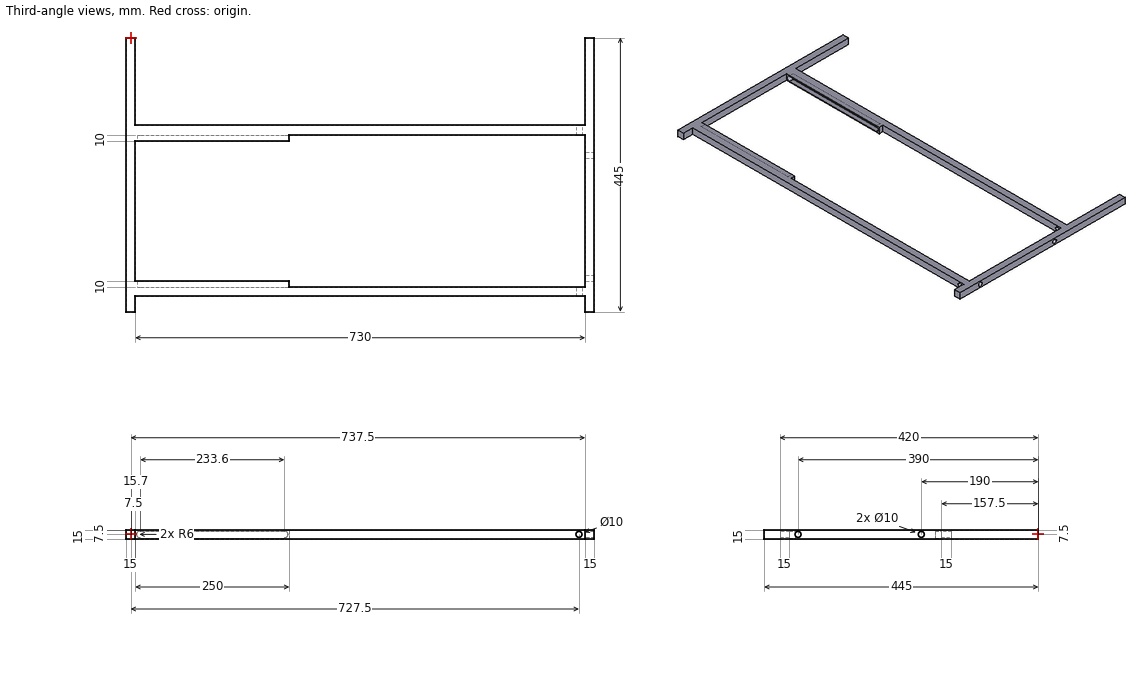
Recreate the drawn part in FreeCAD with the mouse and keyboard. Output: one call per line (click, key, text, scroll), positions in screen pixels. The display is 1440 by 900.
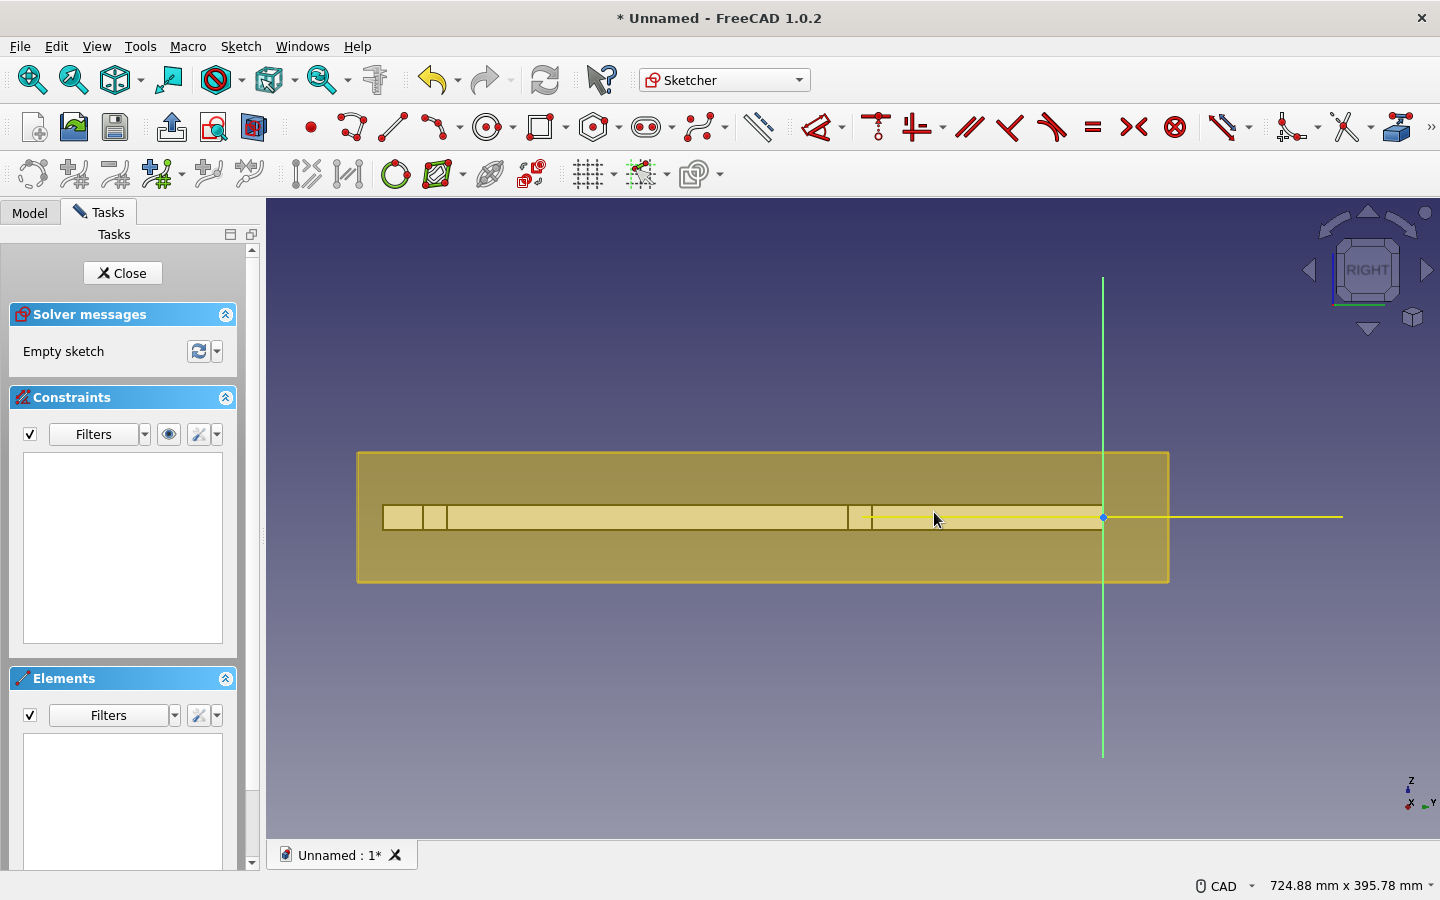
click(486, 128)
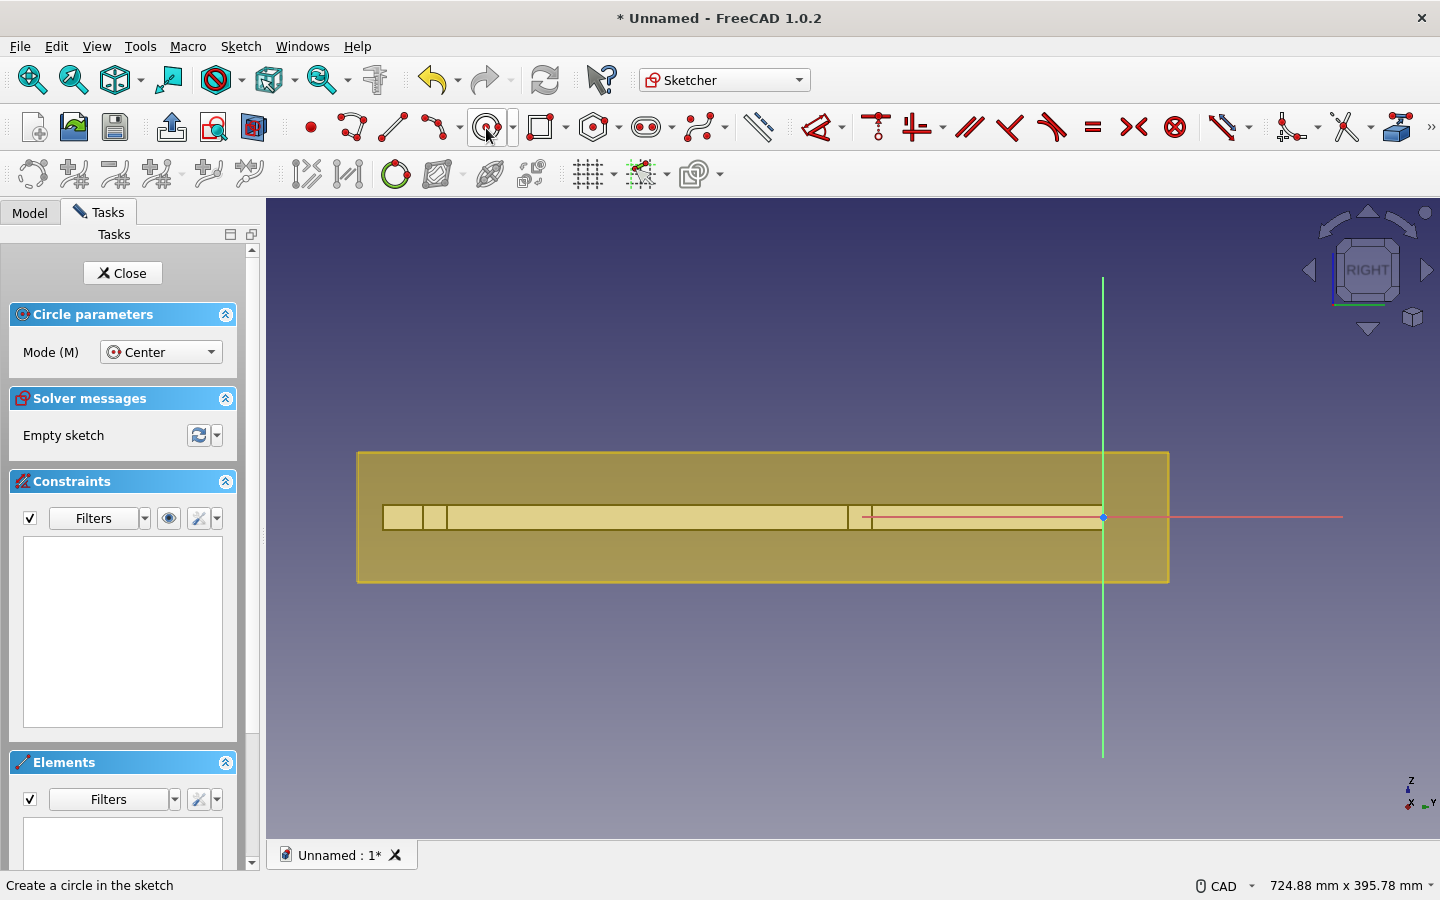
scroll(796, 517, up, 6)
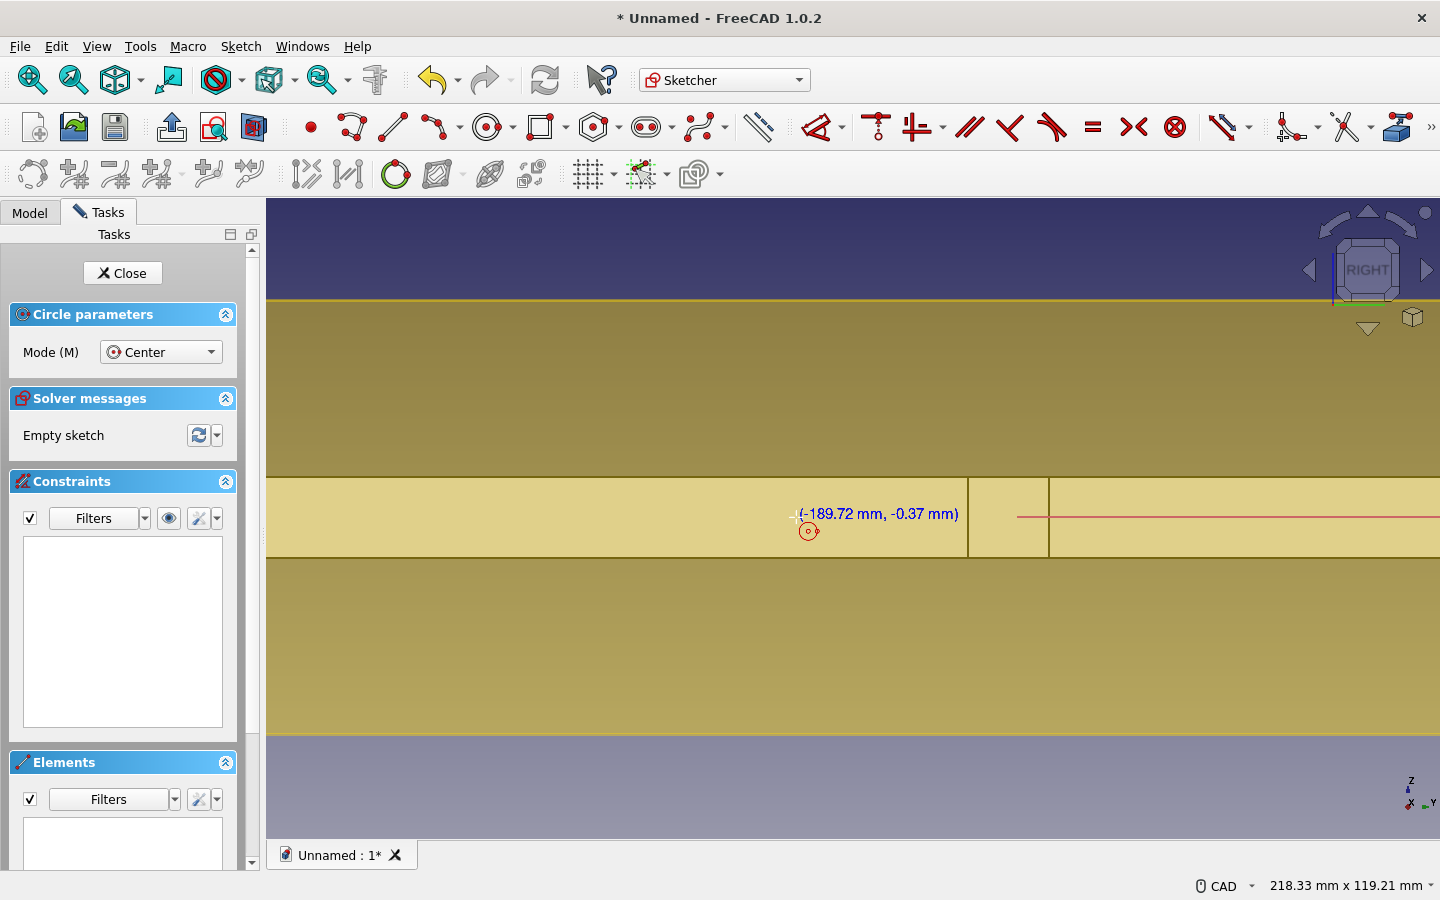
click(793, 517)
click(812, 498)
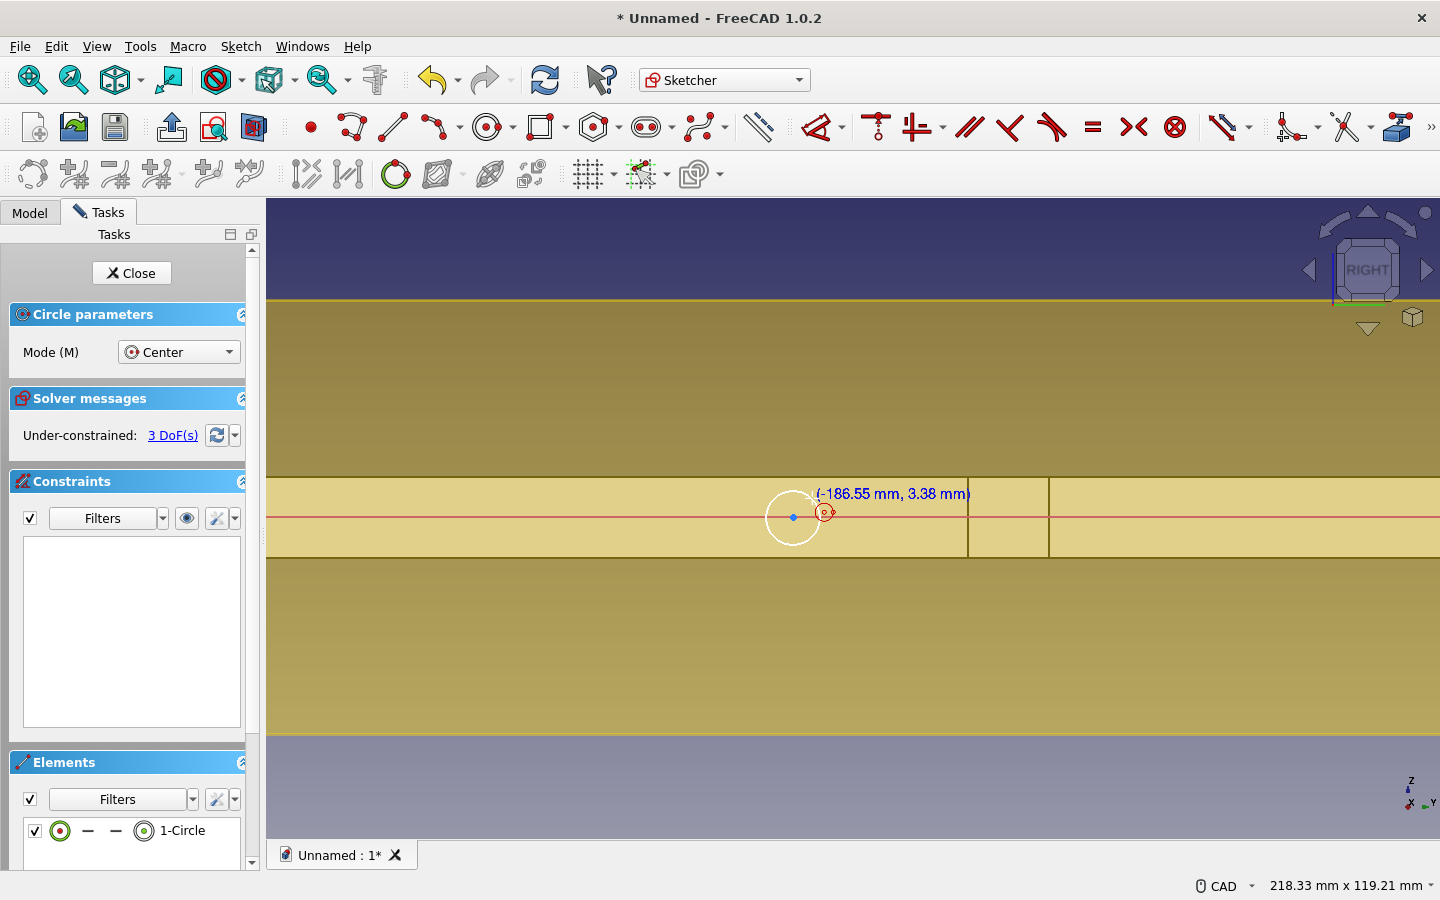
scroll(798, 519, down, 6)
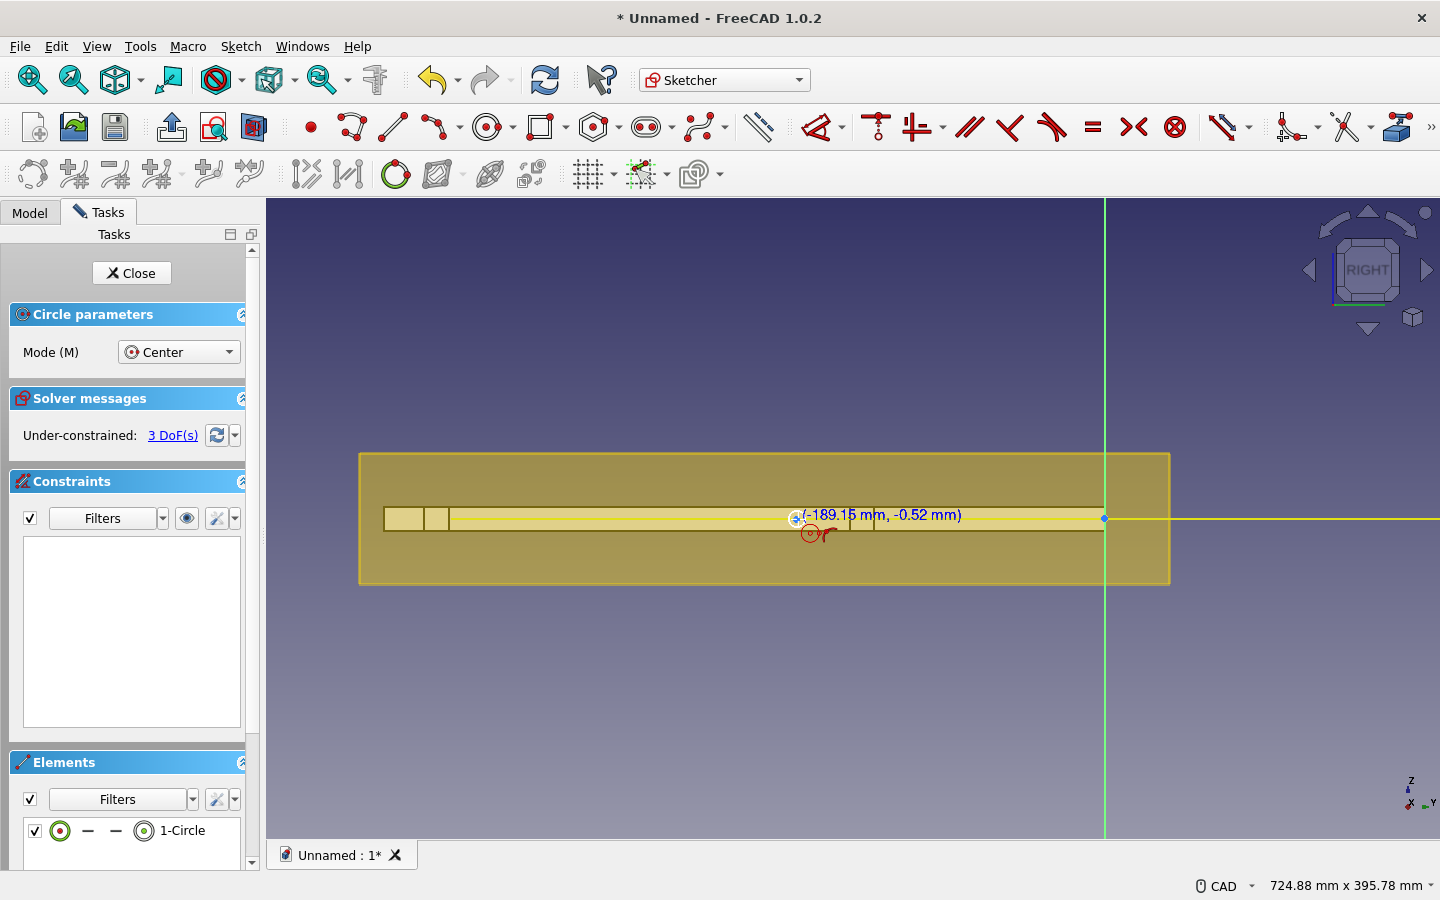
scroll(473, 519, up, 6)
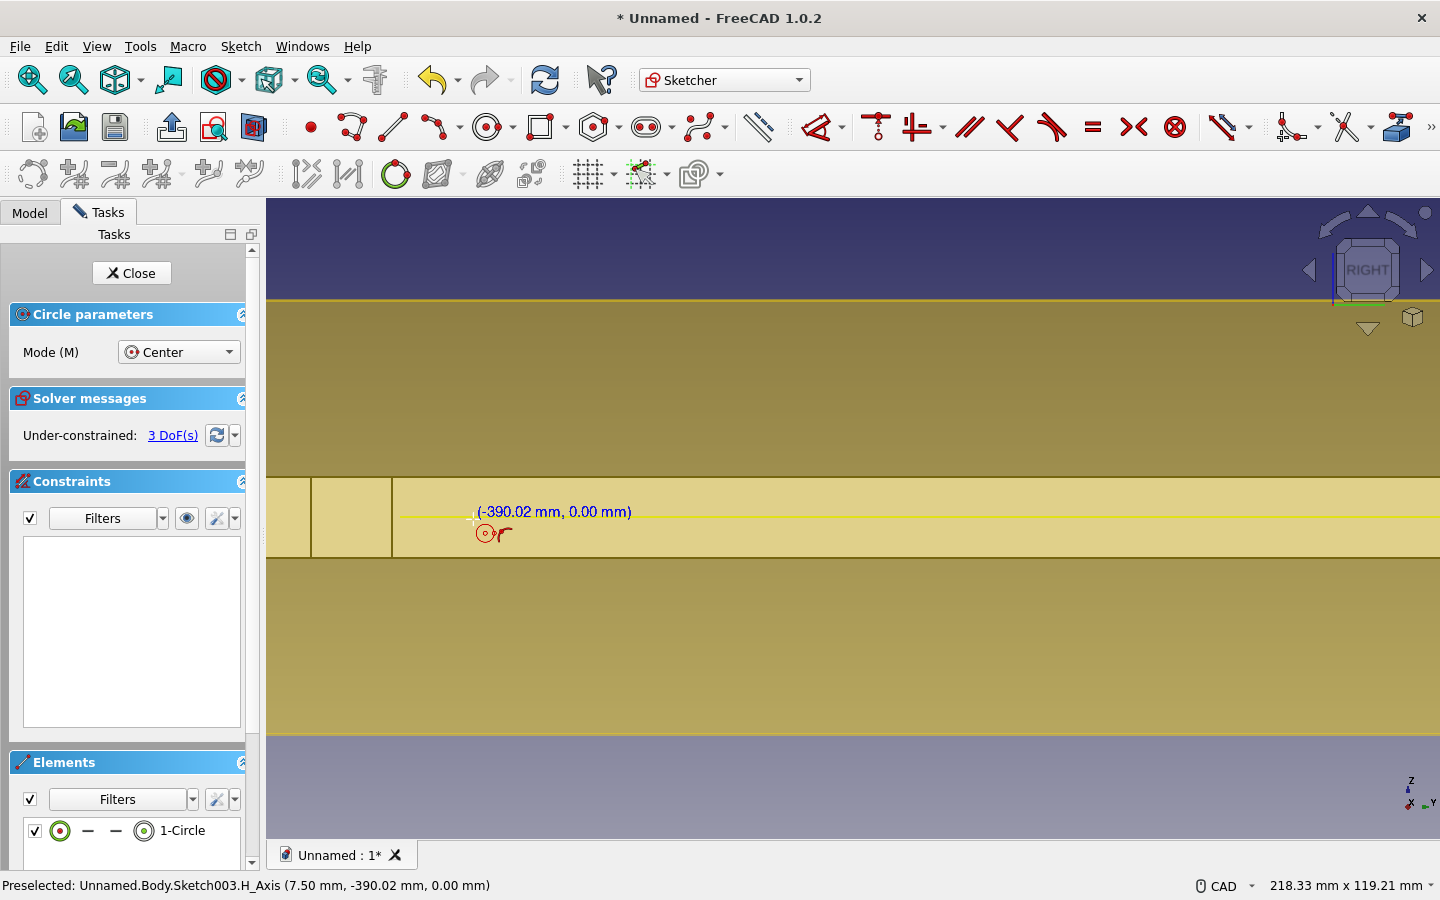
click(473, 517)
click(492, 498)
key(Escape)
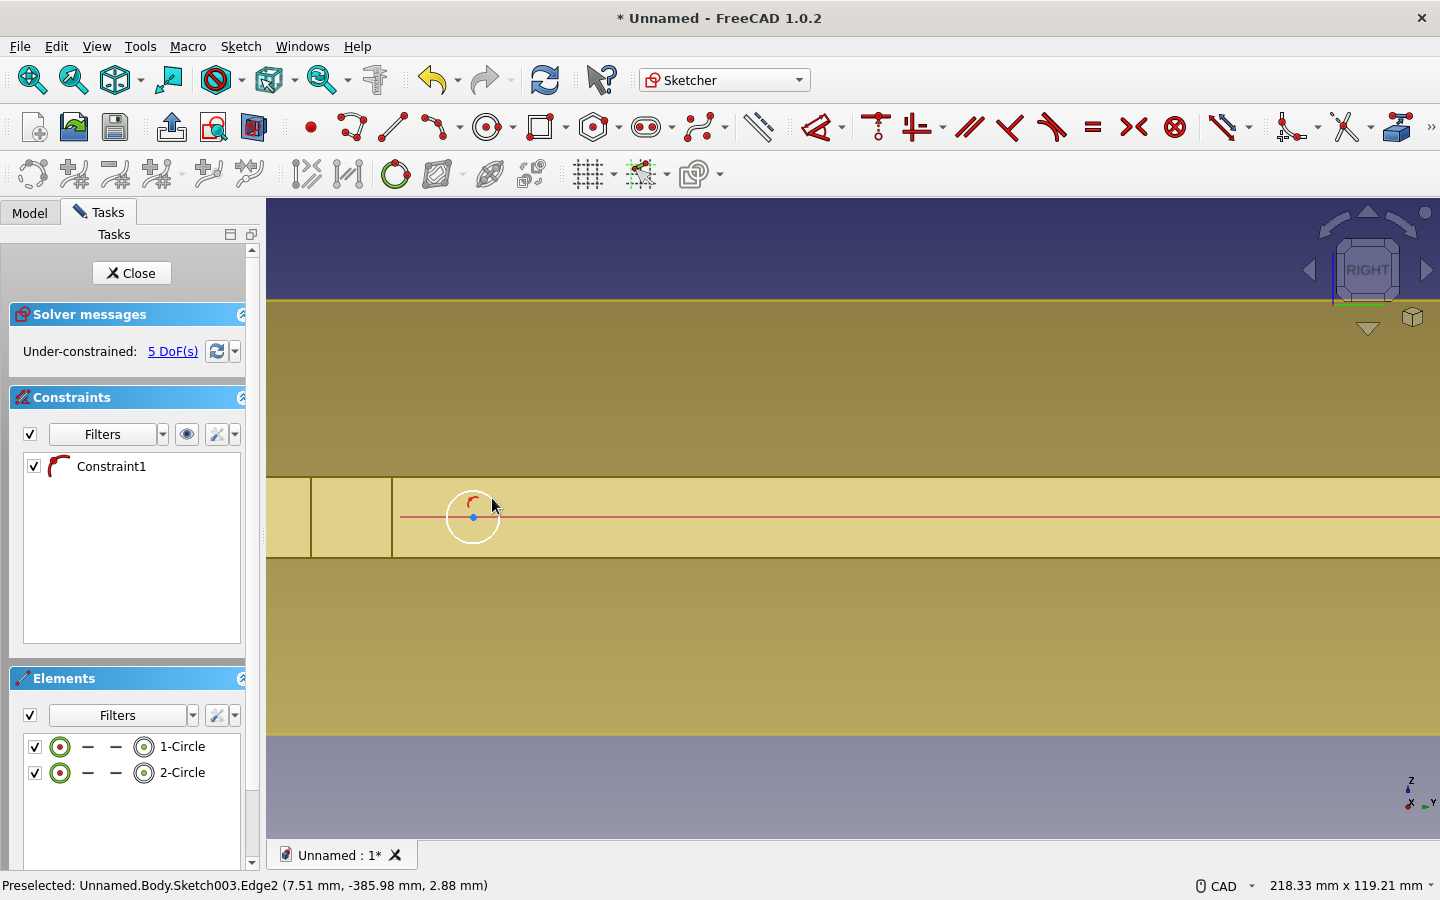
scroll(473, 519, down, 6)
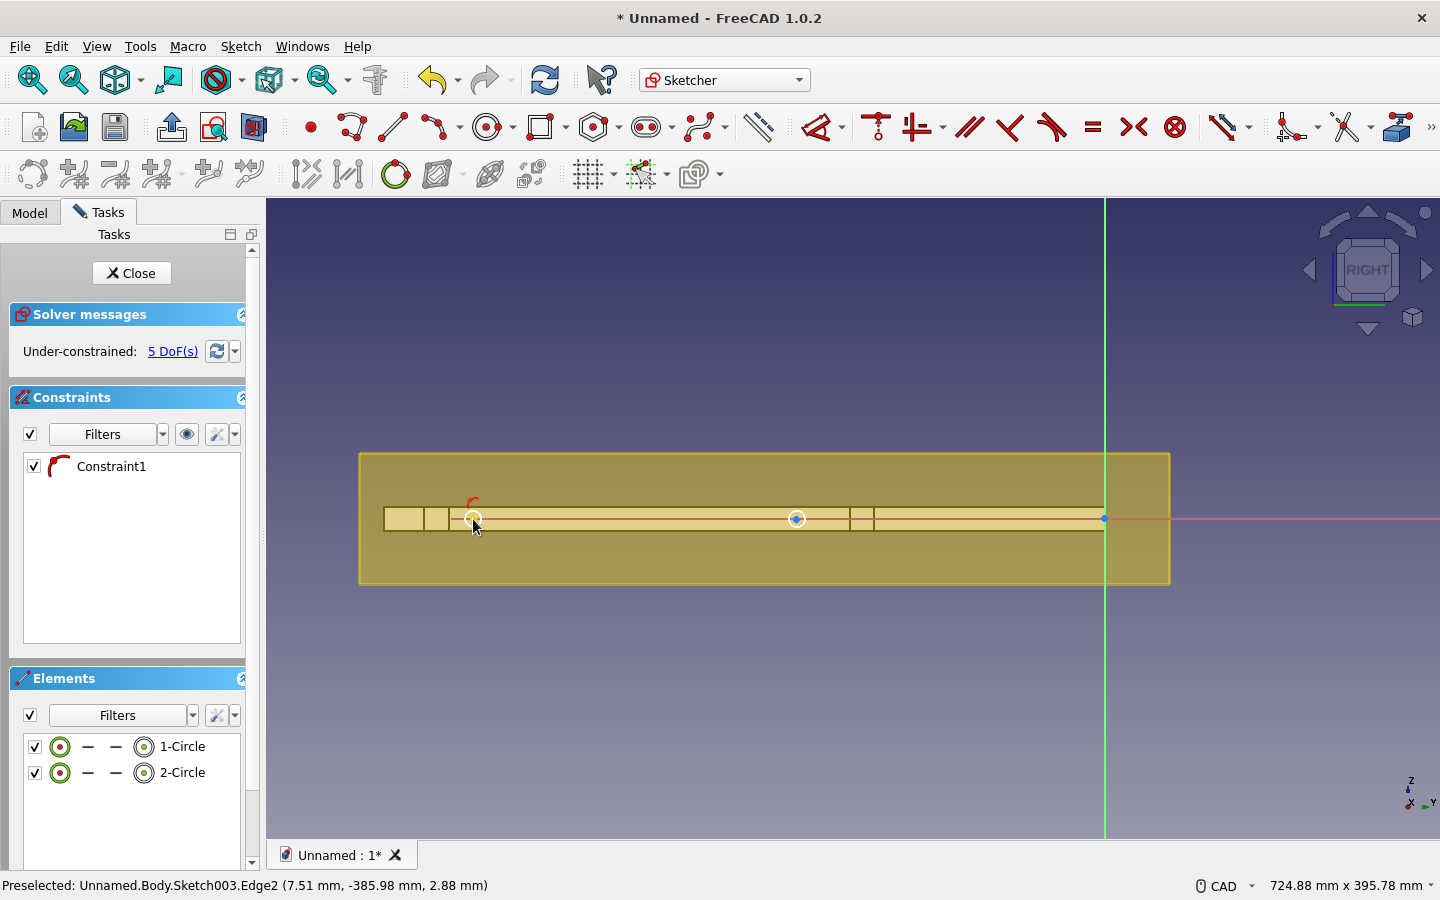
scroll(803, 513, up, 5)